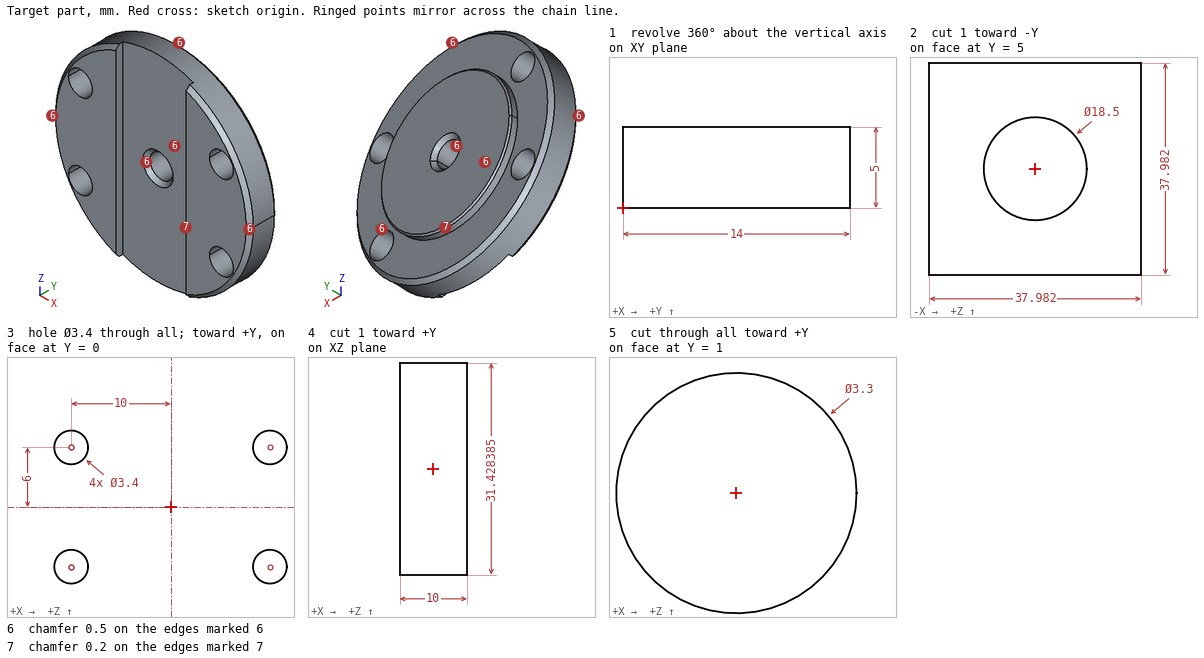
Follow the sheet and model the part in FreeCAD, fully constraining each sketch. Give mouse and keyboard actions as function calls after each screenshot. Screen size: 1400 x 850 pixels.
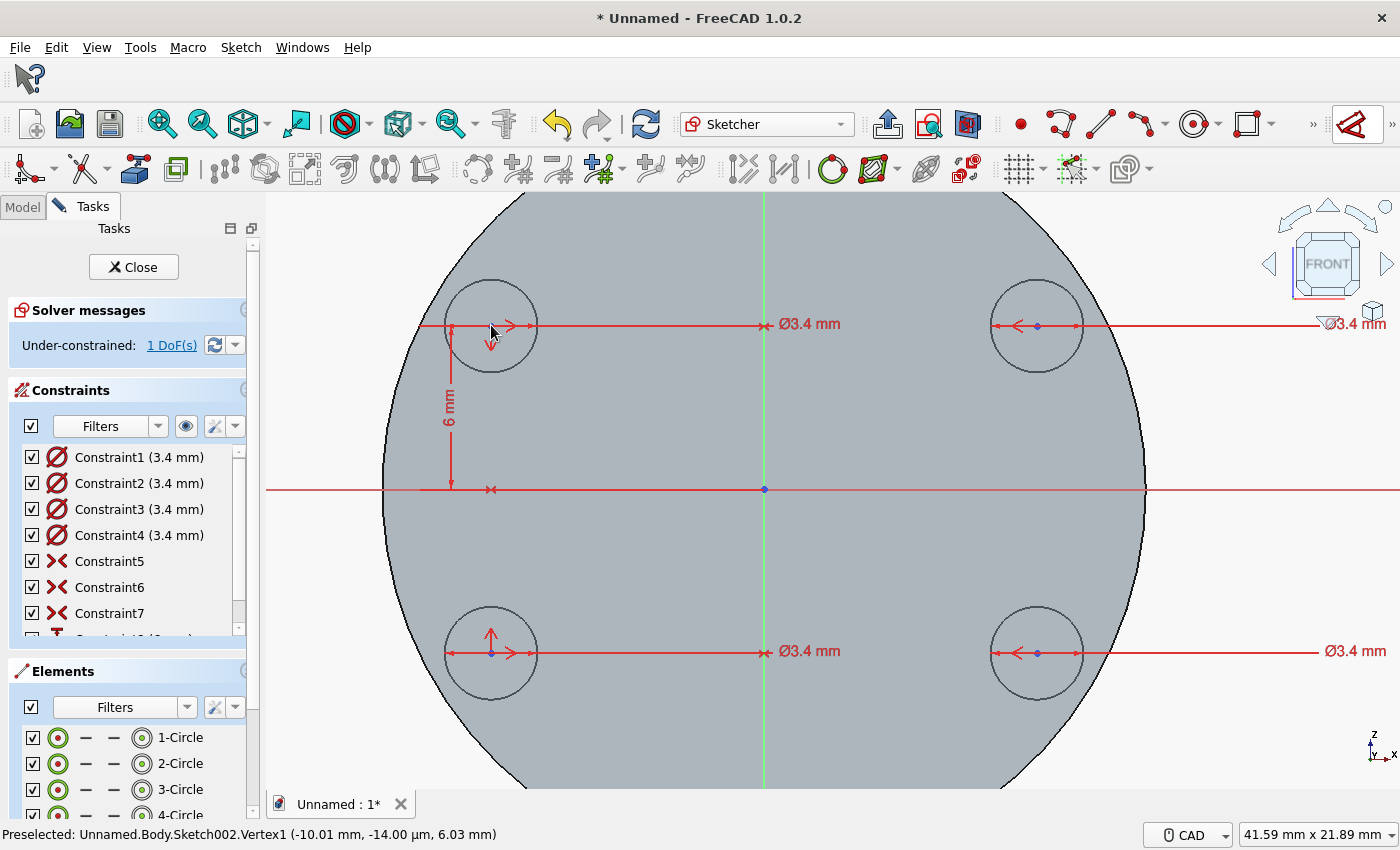
click(491, 326)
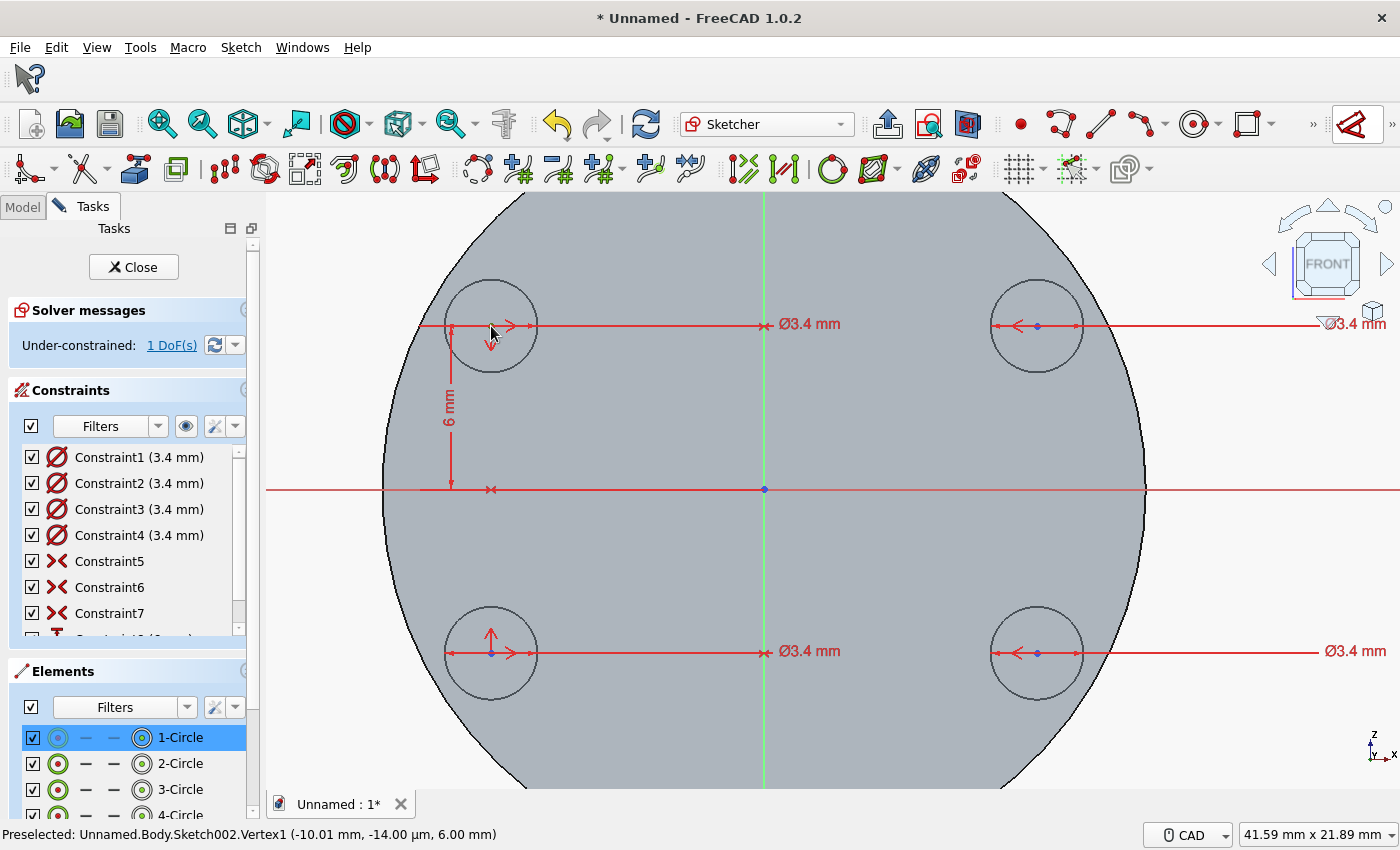
key(l)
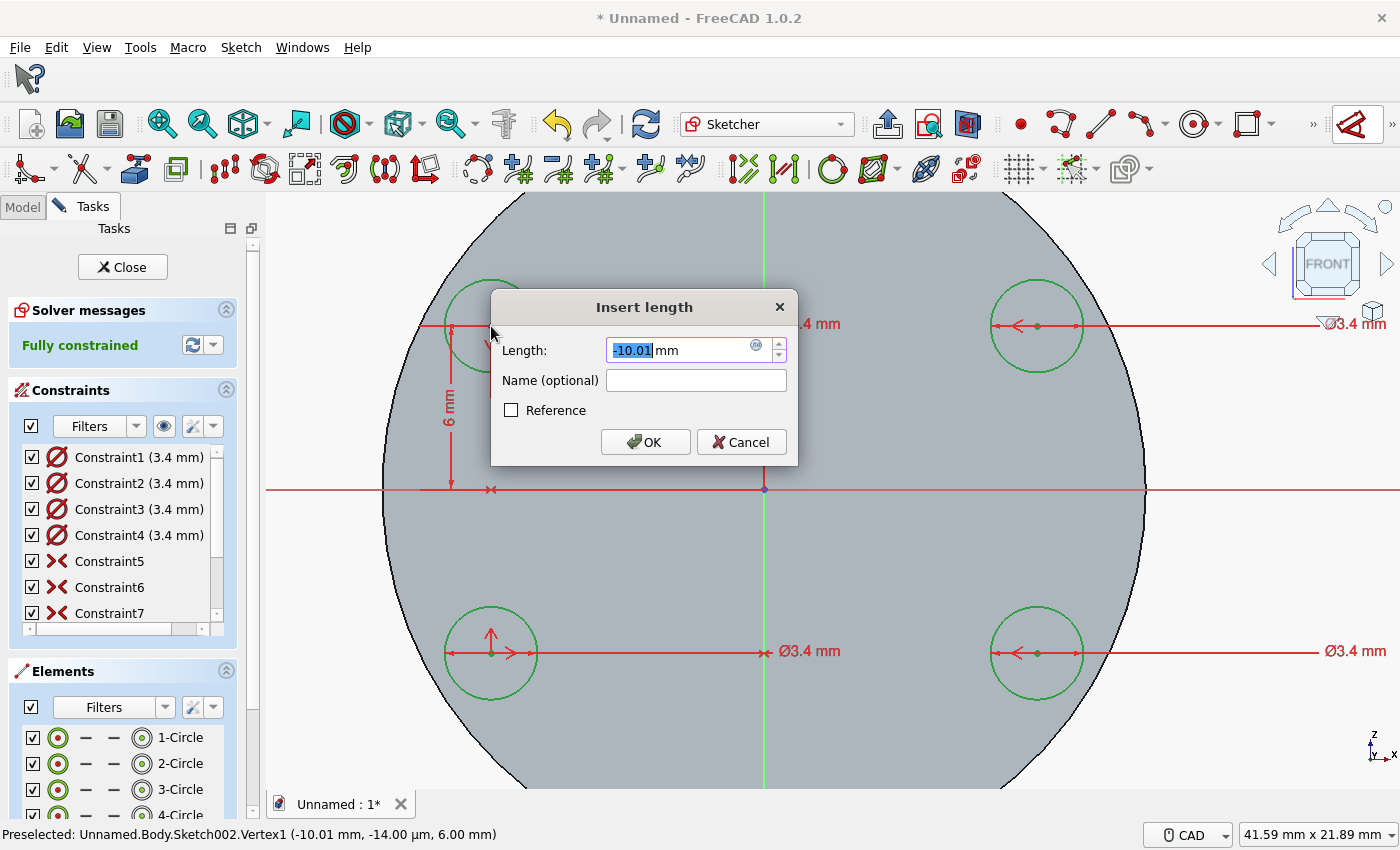
text(-10)
key(Return)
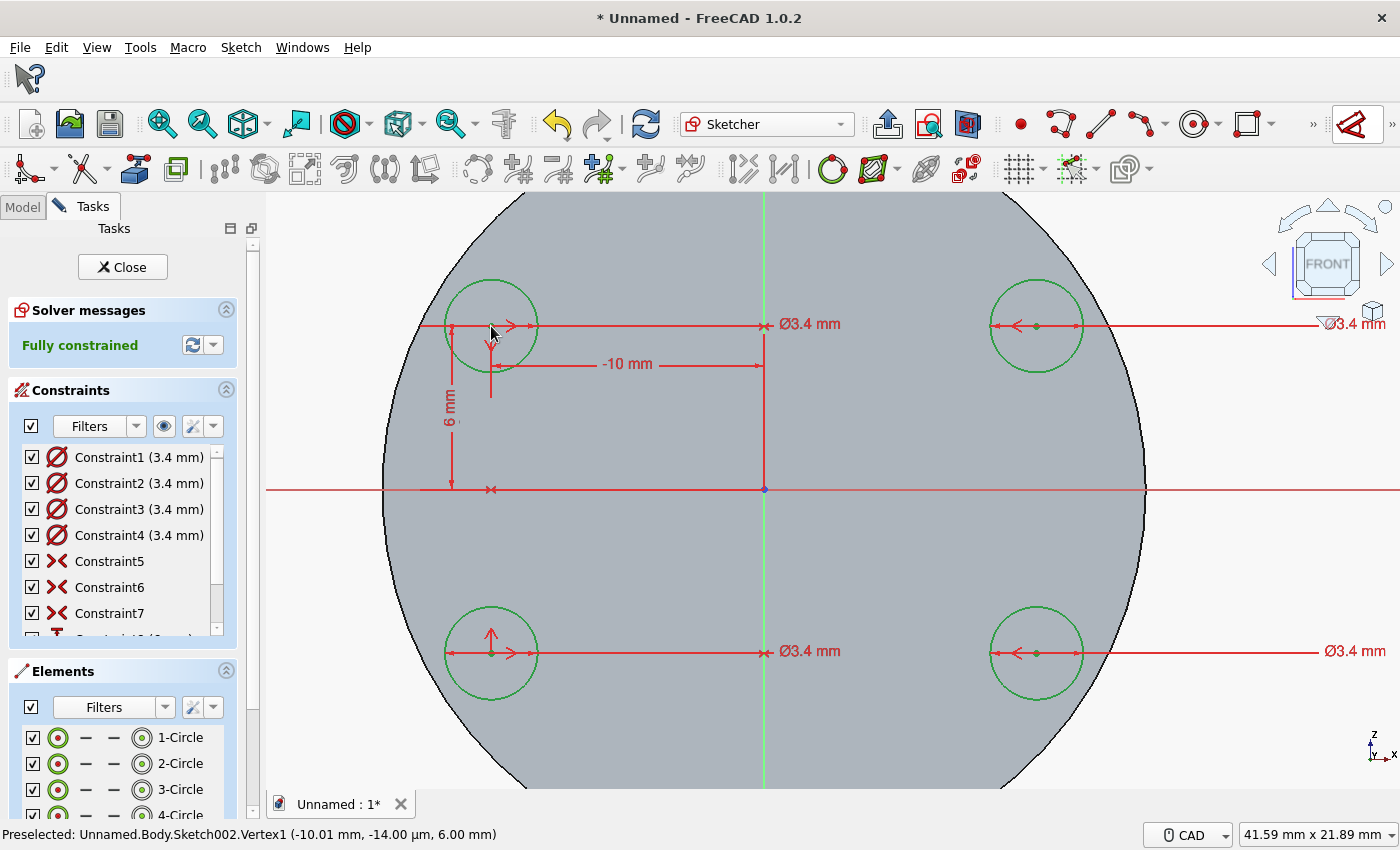
click(123, 267)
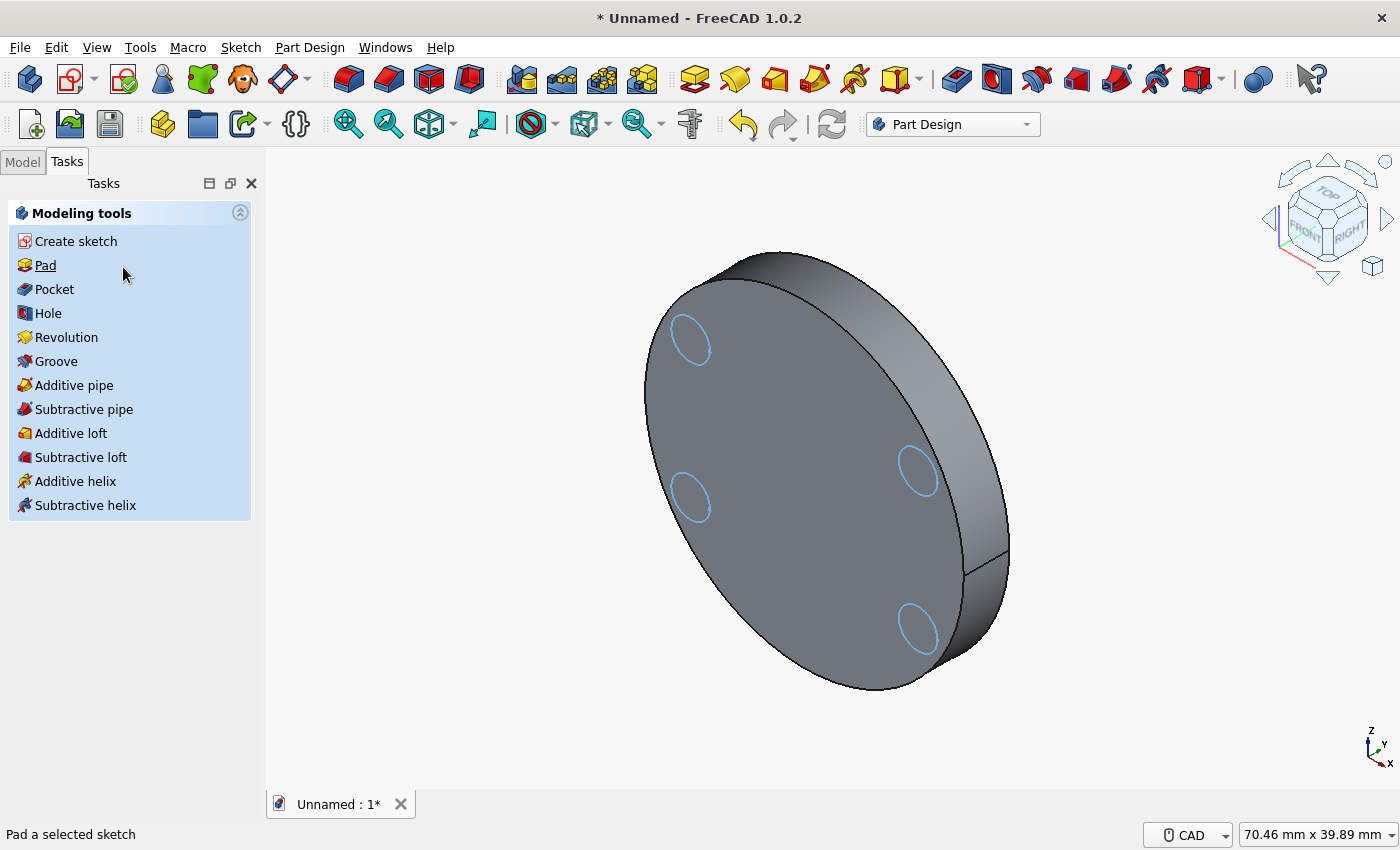
click(998, 80)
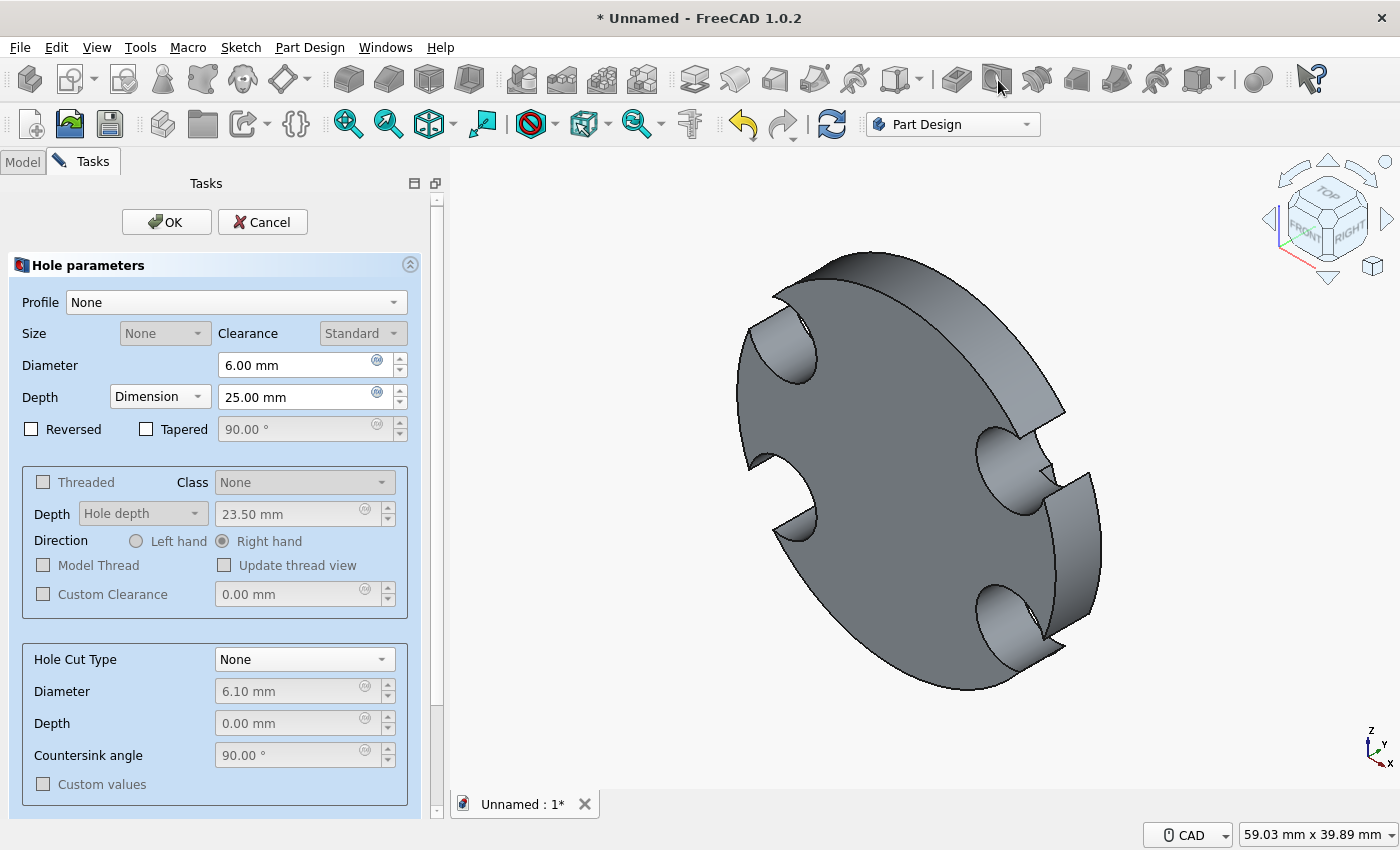
triple_click(305, 365)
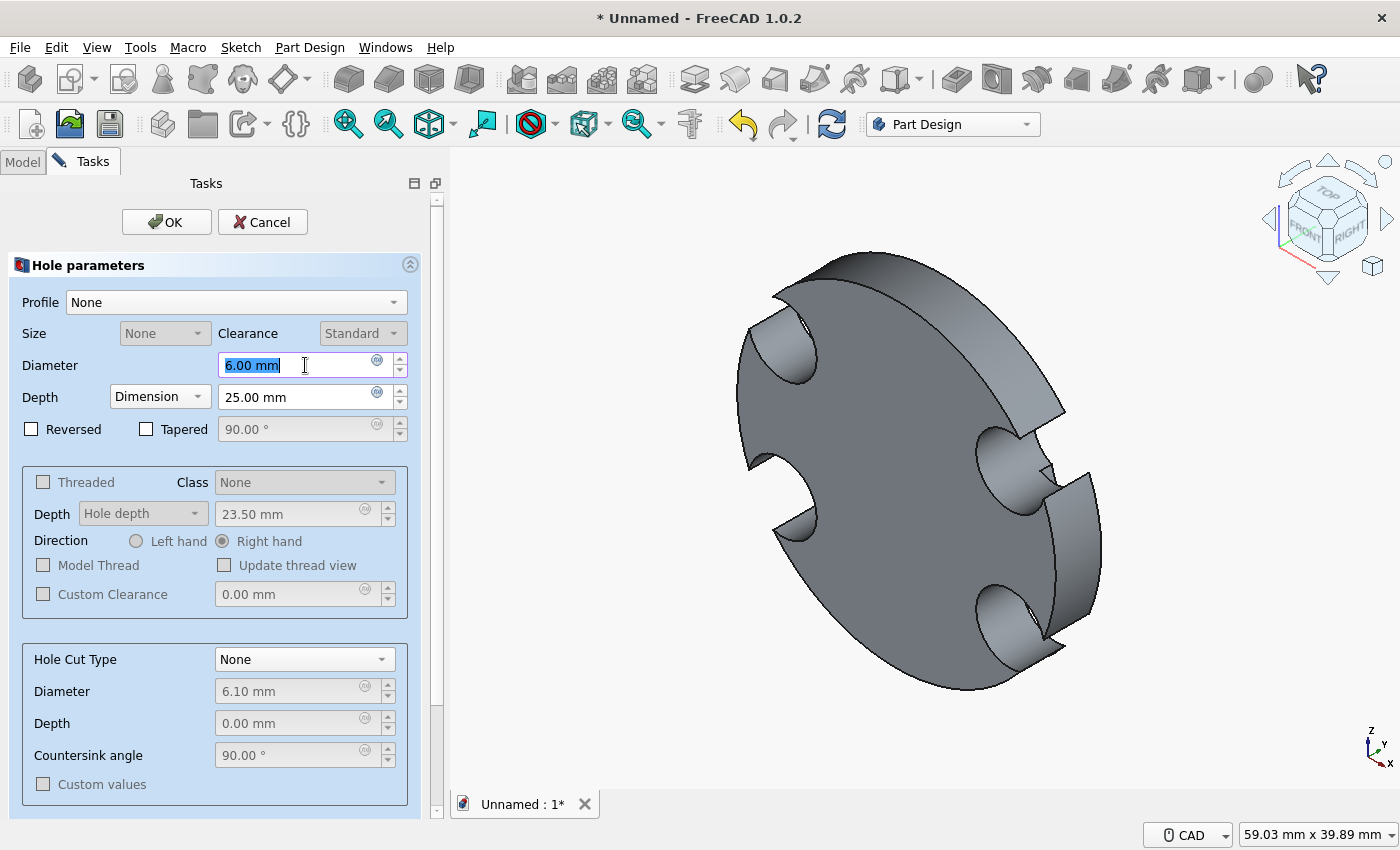
text(3.4)
key(Tab)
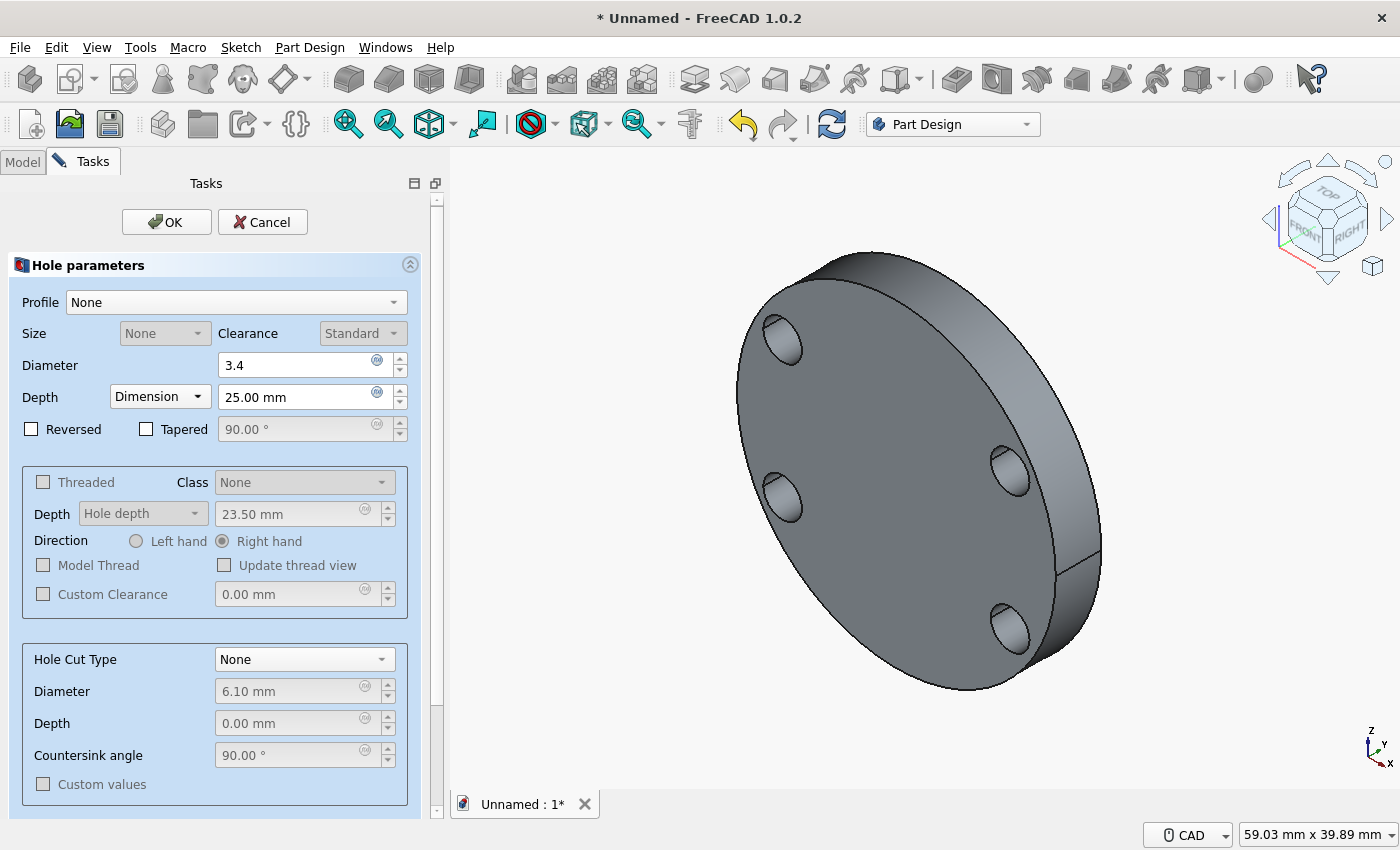
click(161, 396)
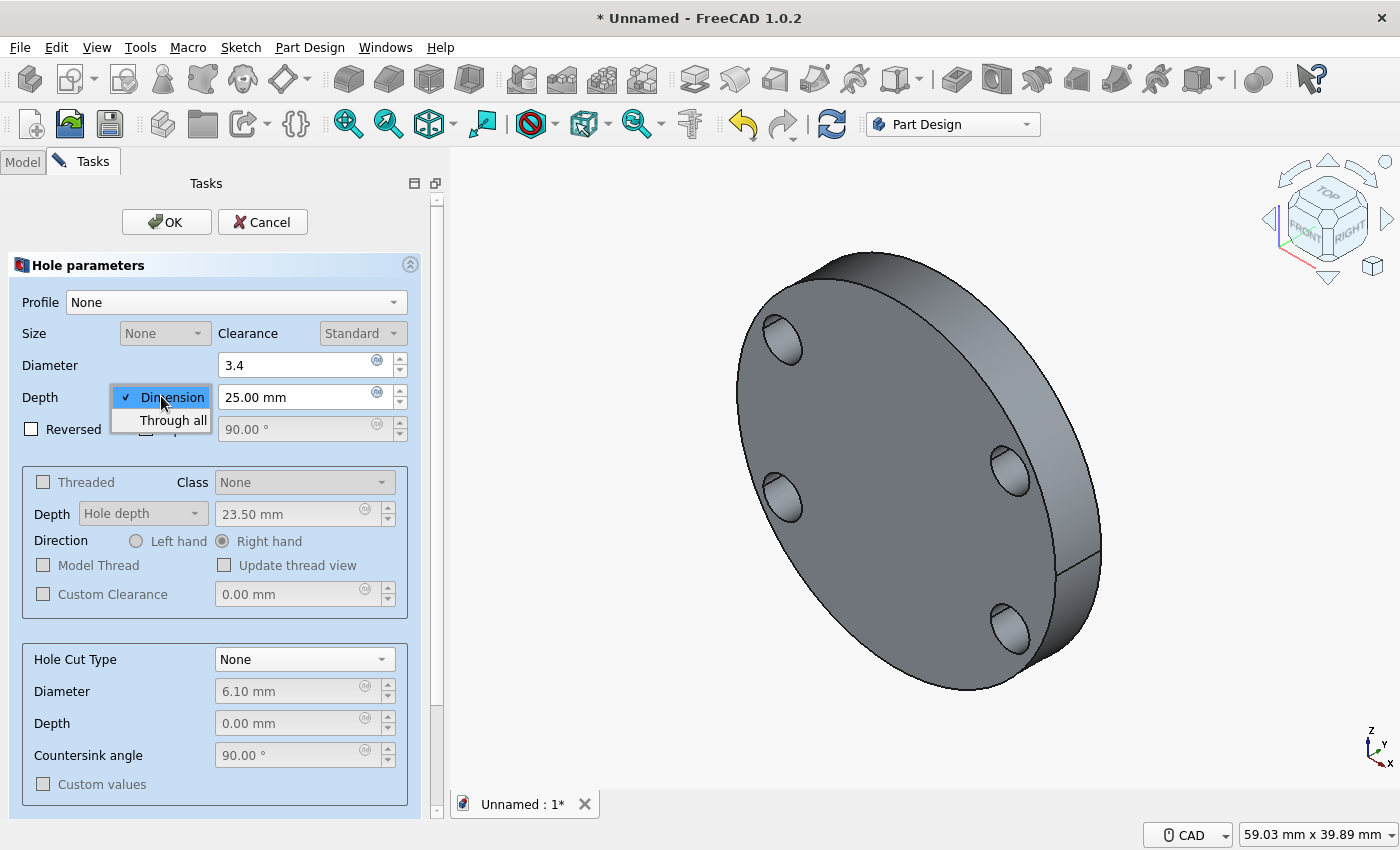
click(160, 420)